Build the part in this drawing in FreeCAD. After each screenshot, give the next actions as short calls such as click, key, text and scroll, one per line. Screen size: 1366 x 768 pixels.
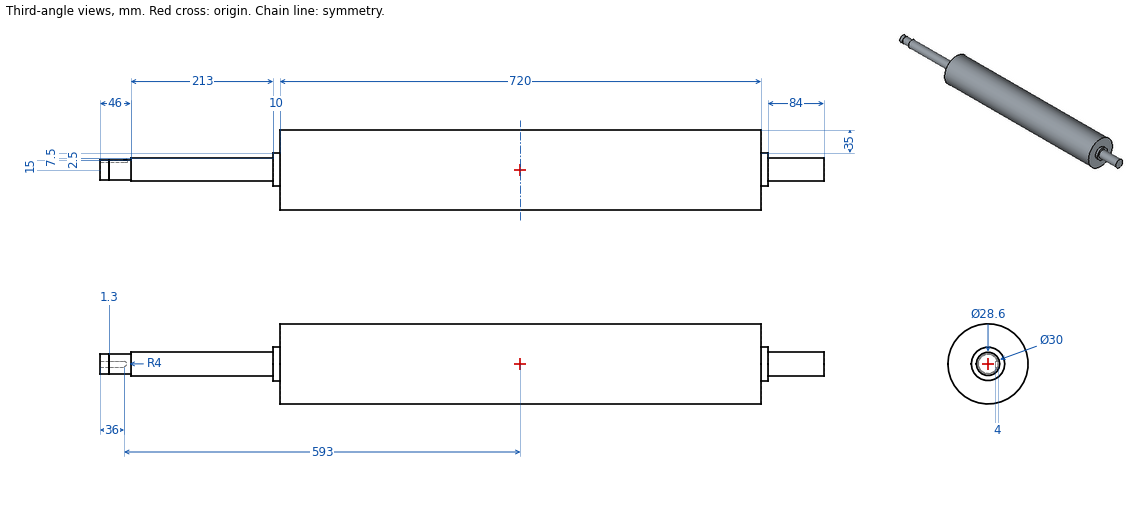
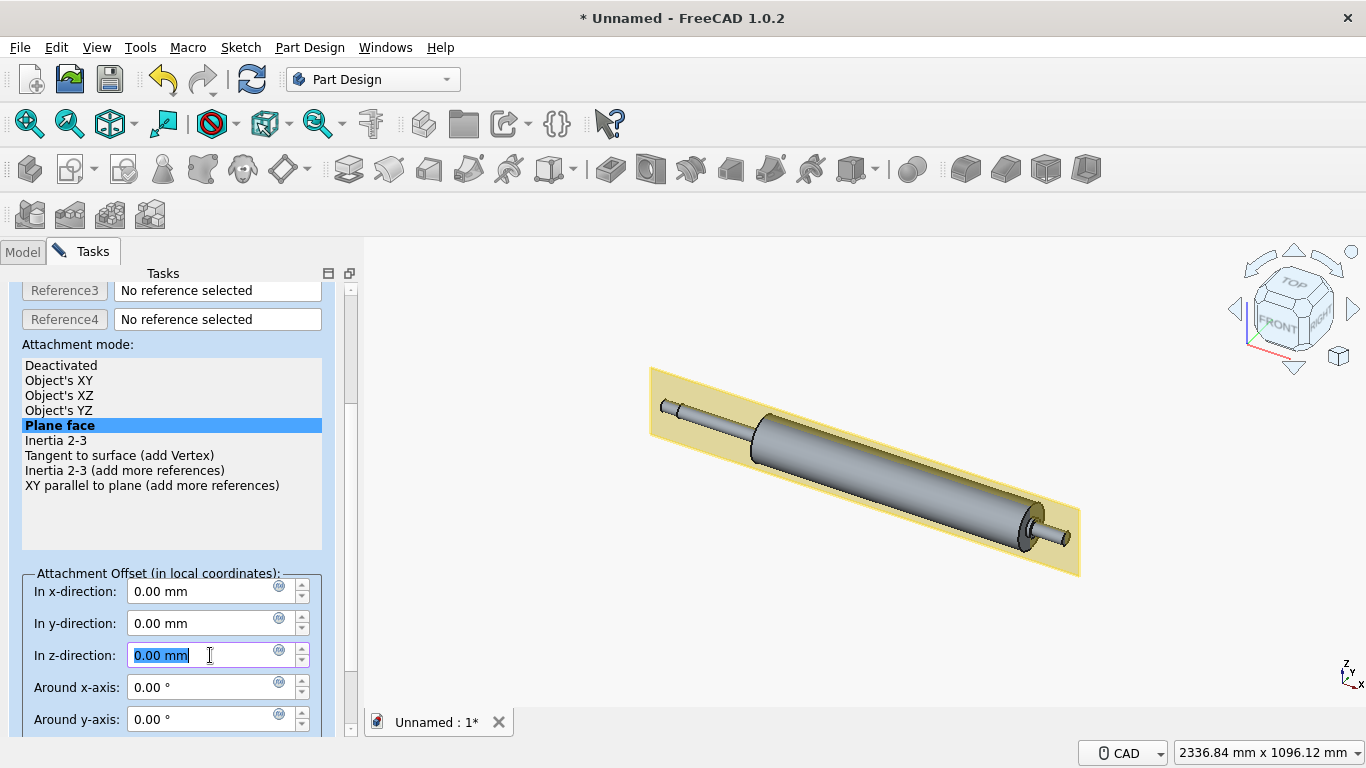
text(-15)
key(Tab)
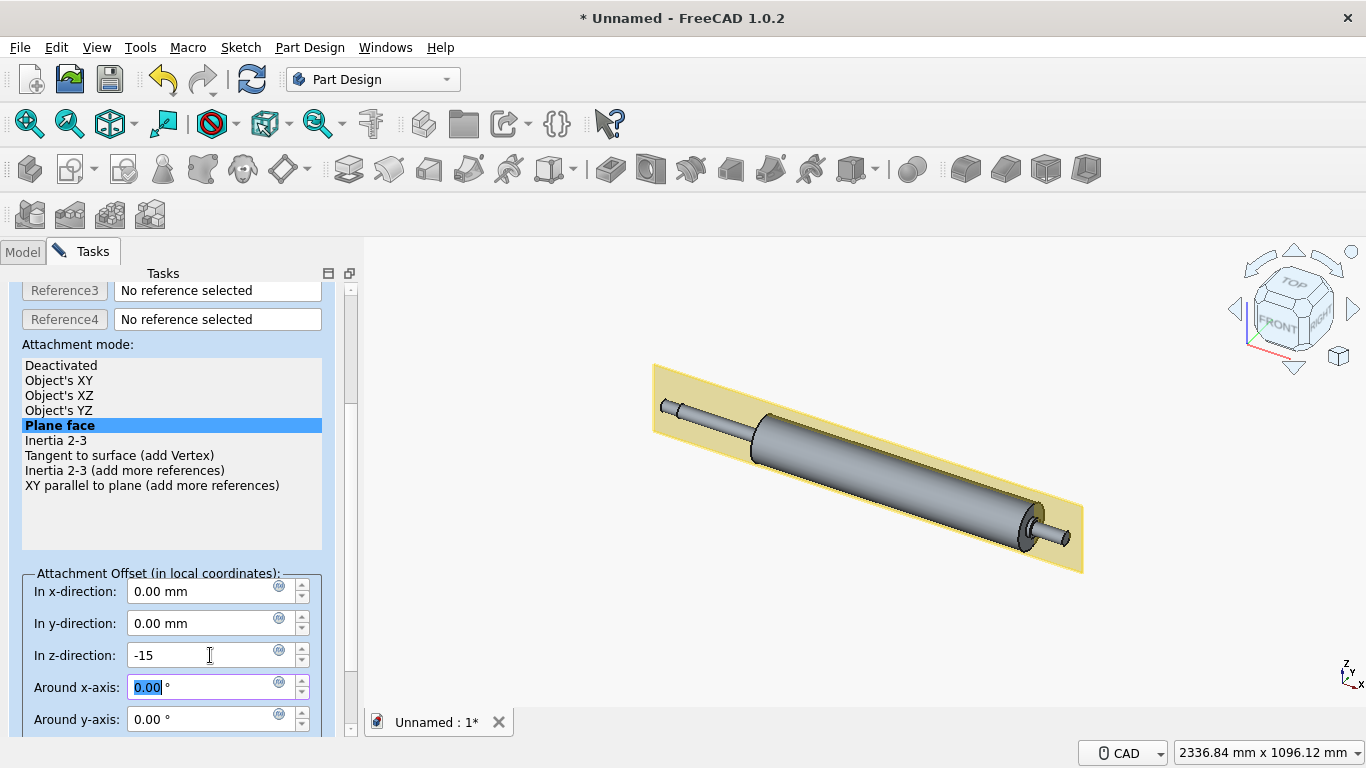
scroll(351, 510, up, 4)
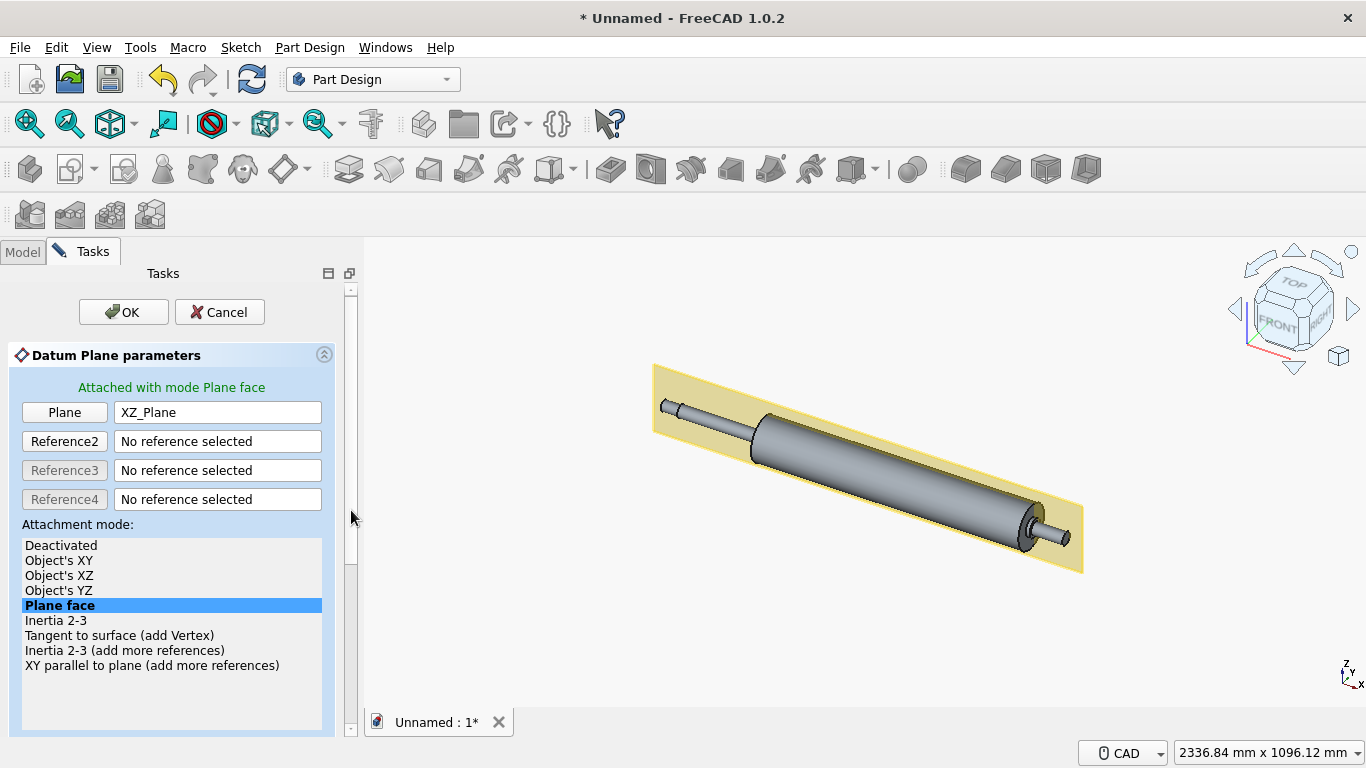
click(124, 312)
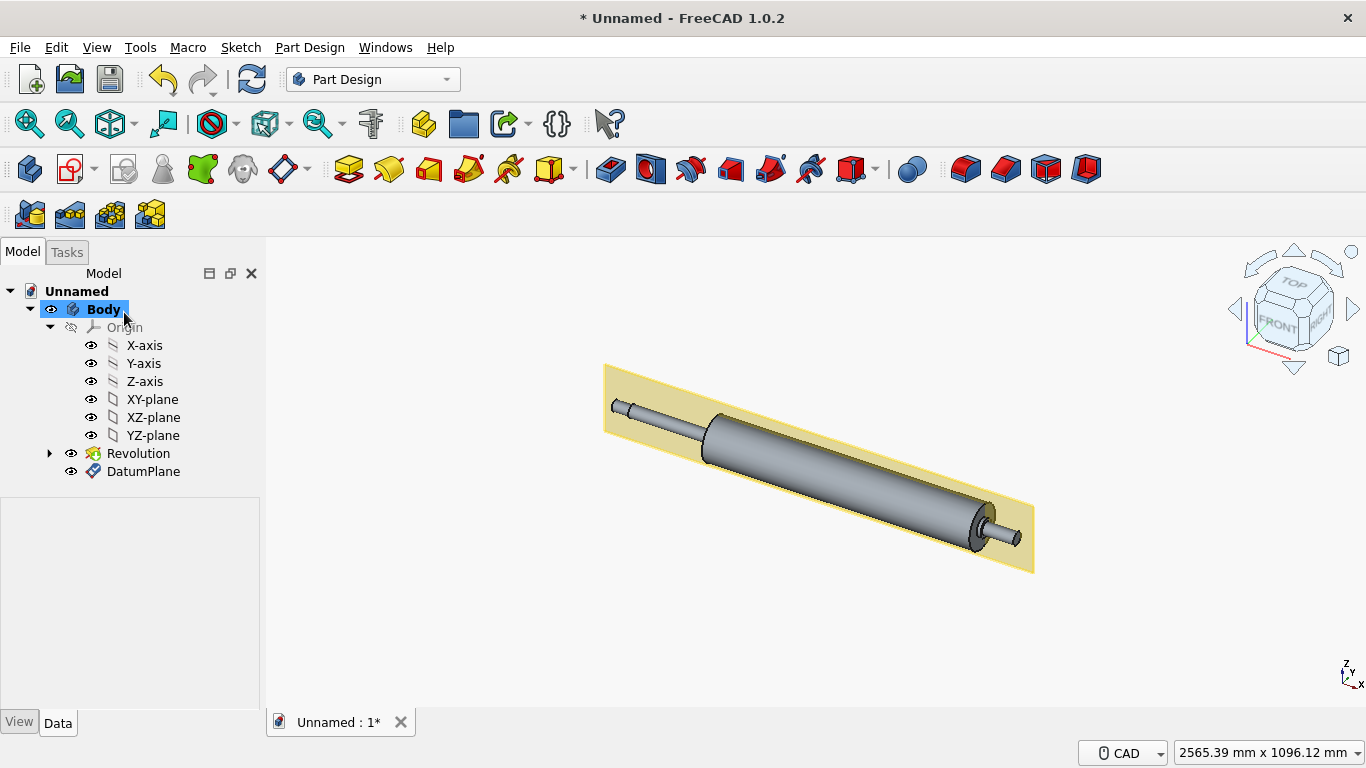
click(116, 471)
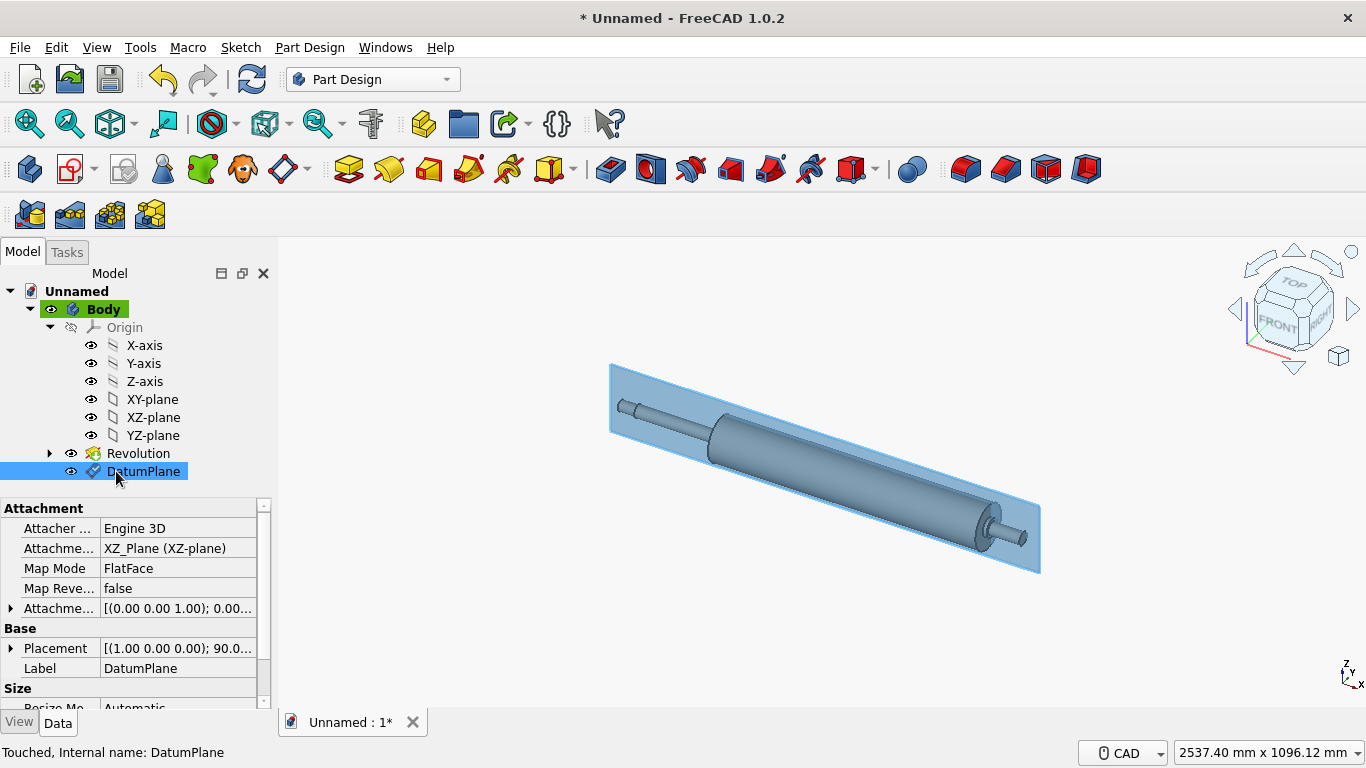
click(70, 170)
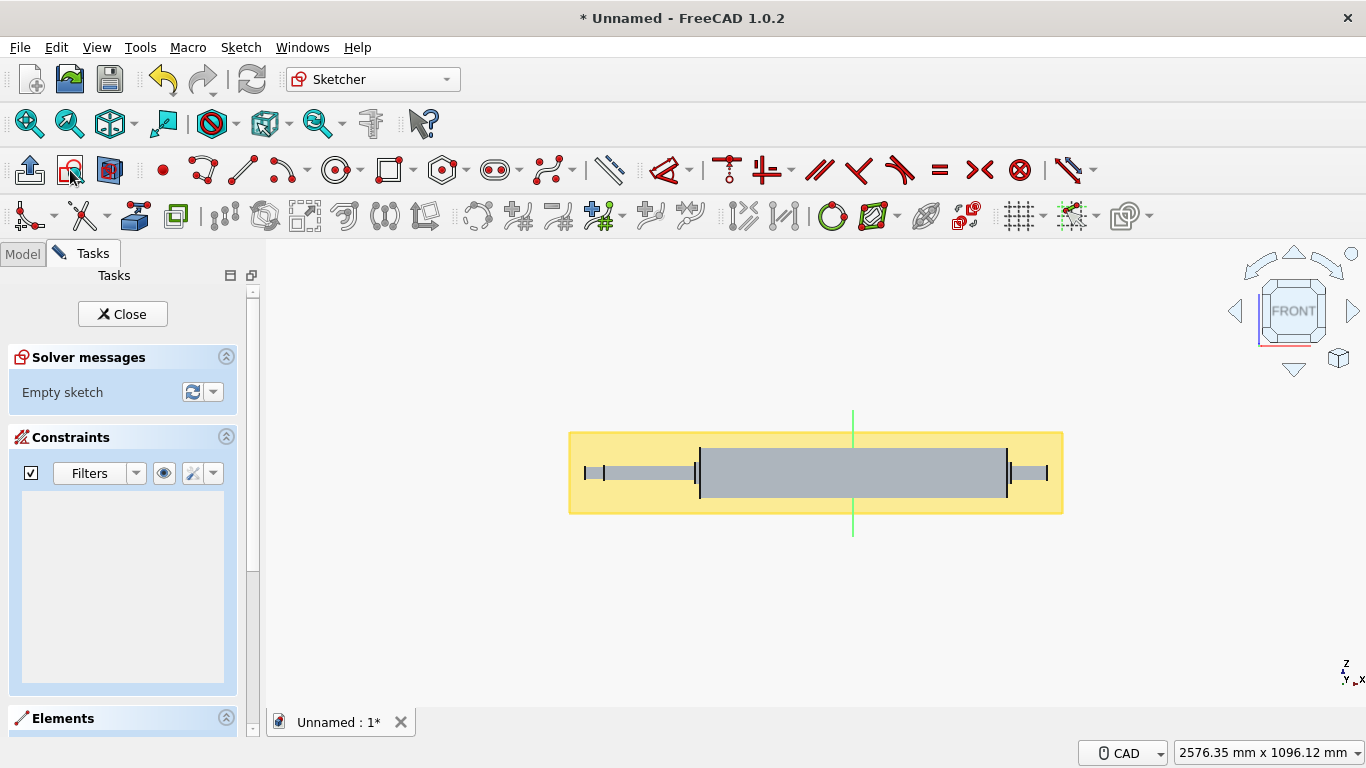
click(110, 170)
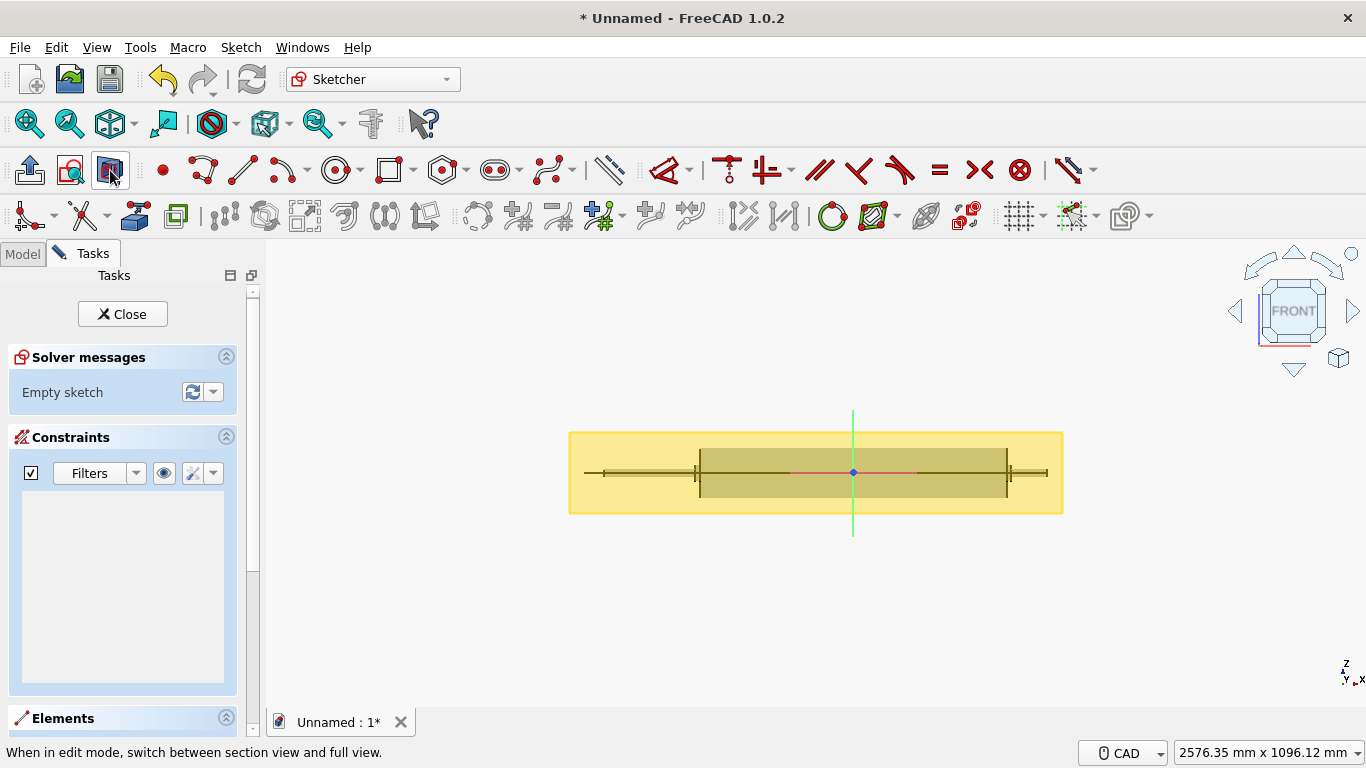
scroll(585, 473, up, 15)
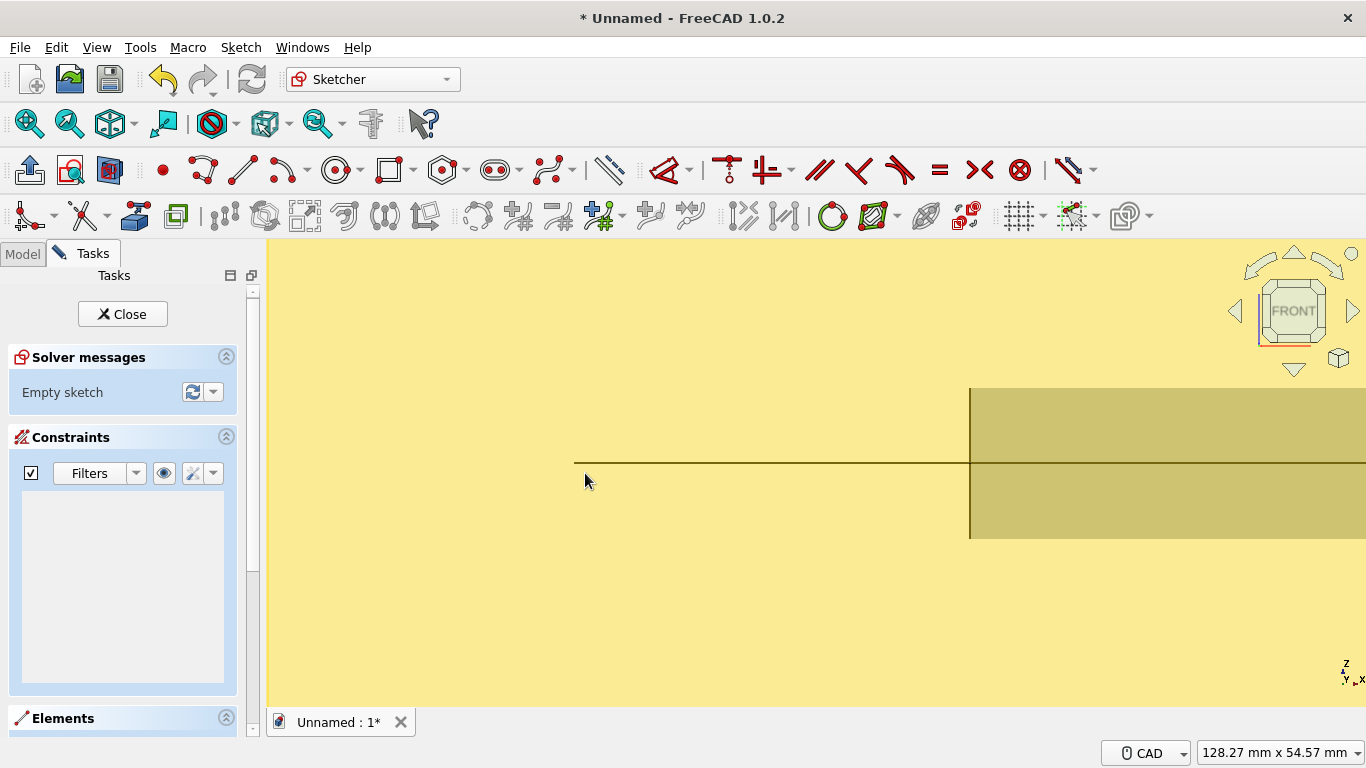
scroll(746, 452, up, 3)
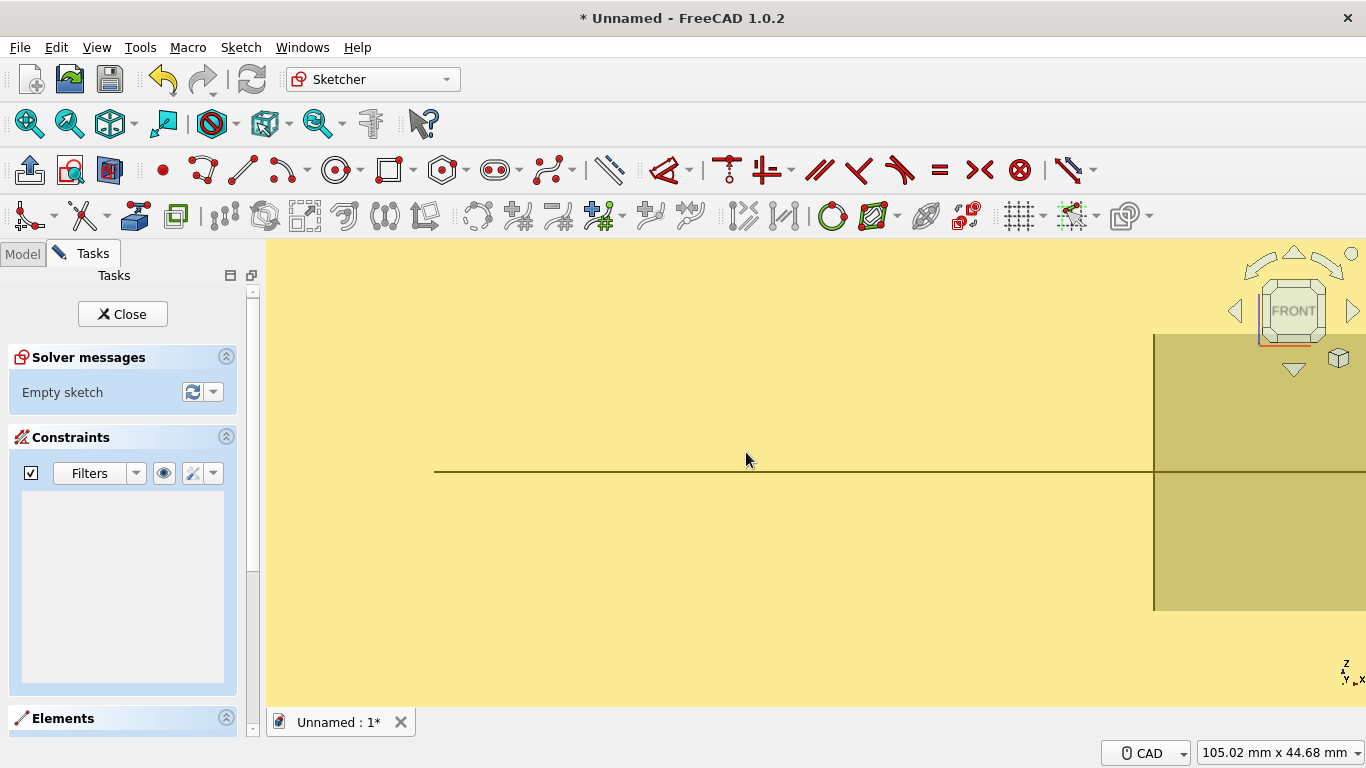
click(204, 170)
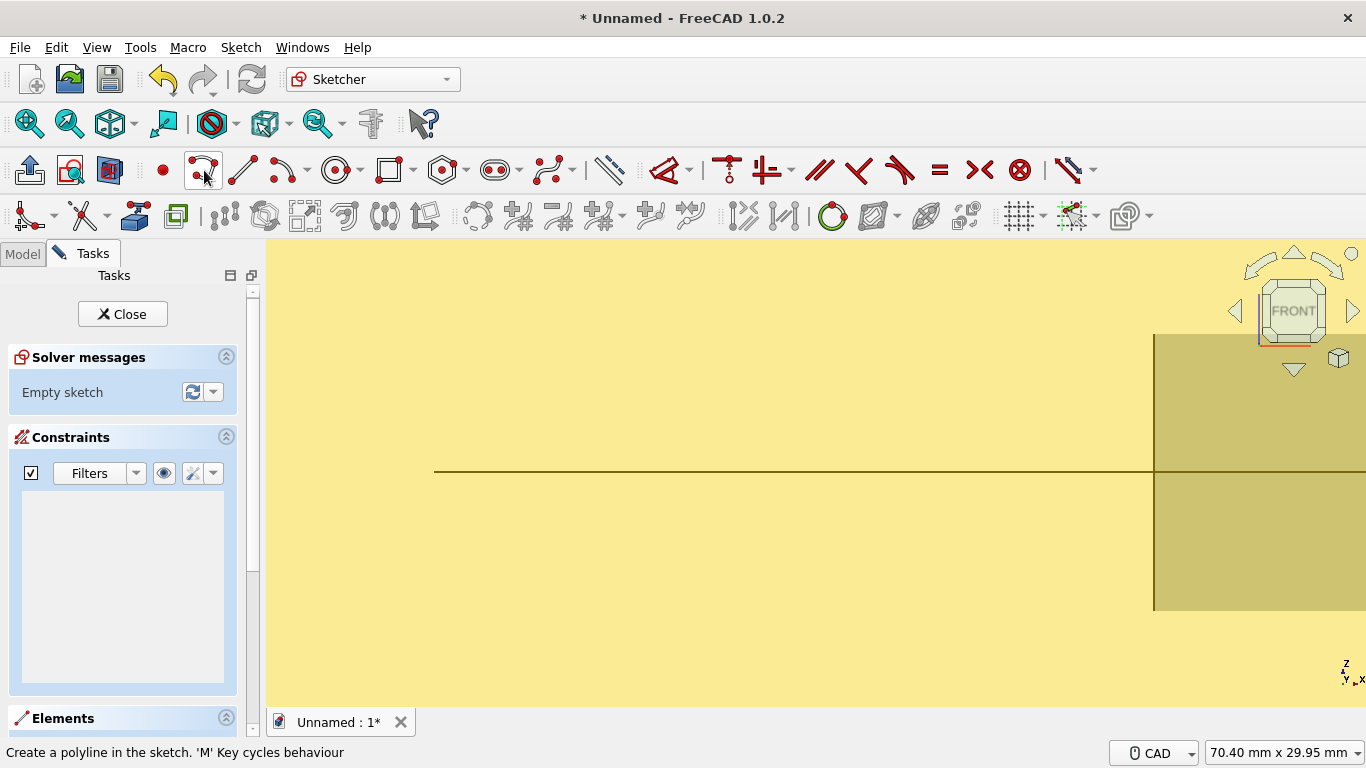
click(997, 535)
click(435, 535)
click(435, 410)
click(997, 410)
right_click(997, 410)